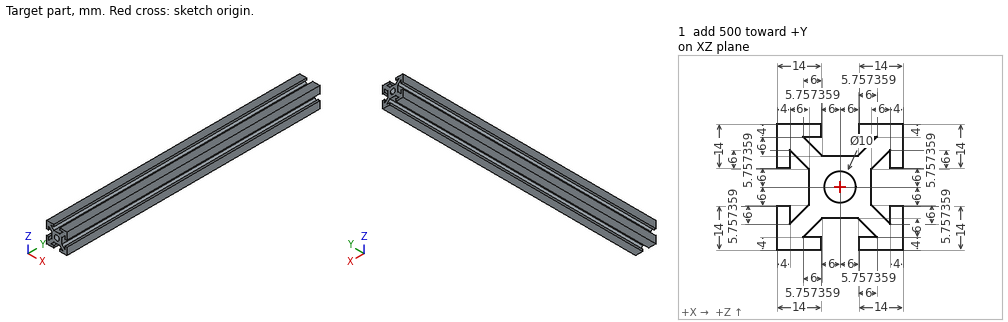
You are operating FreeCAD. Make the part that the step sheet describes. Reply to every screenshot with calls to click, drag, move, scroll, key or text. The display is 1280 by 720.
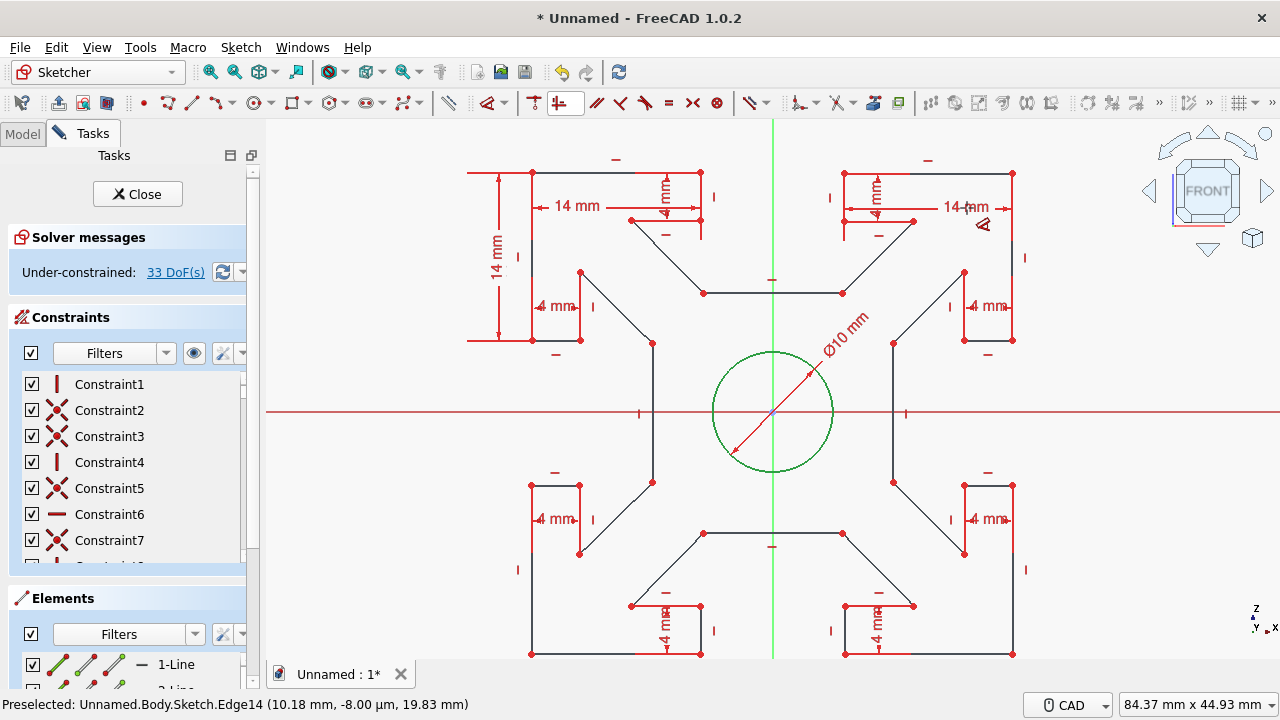
click(1012, 224)
click(1046, 257)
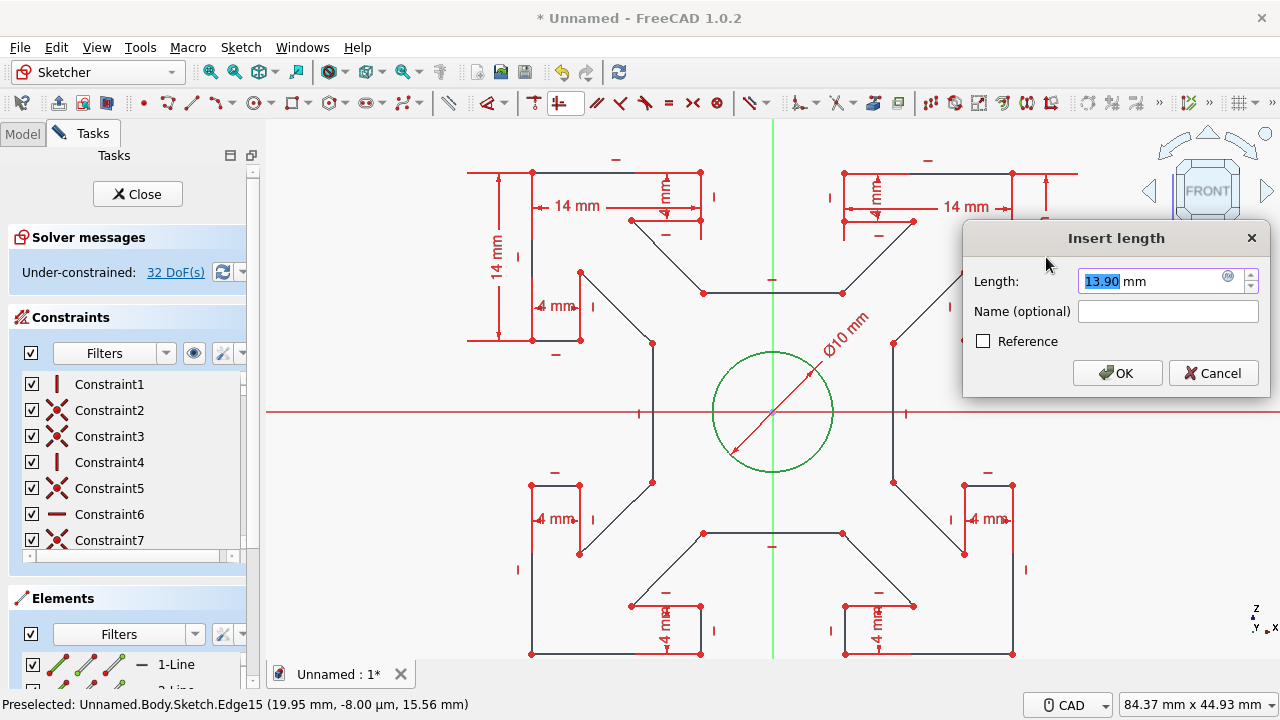
text(14)
key(Return)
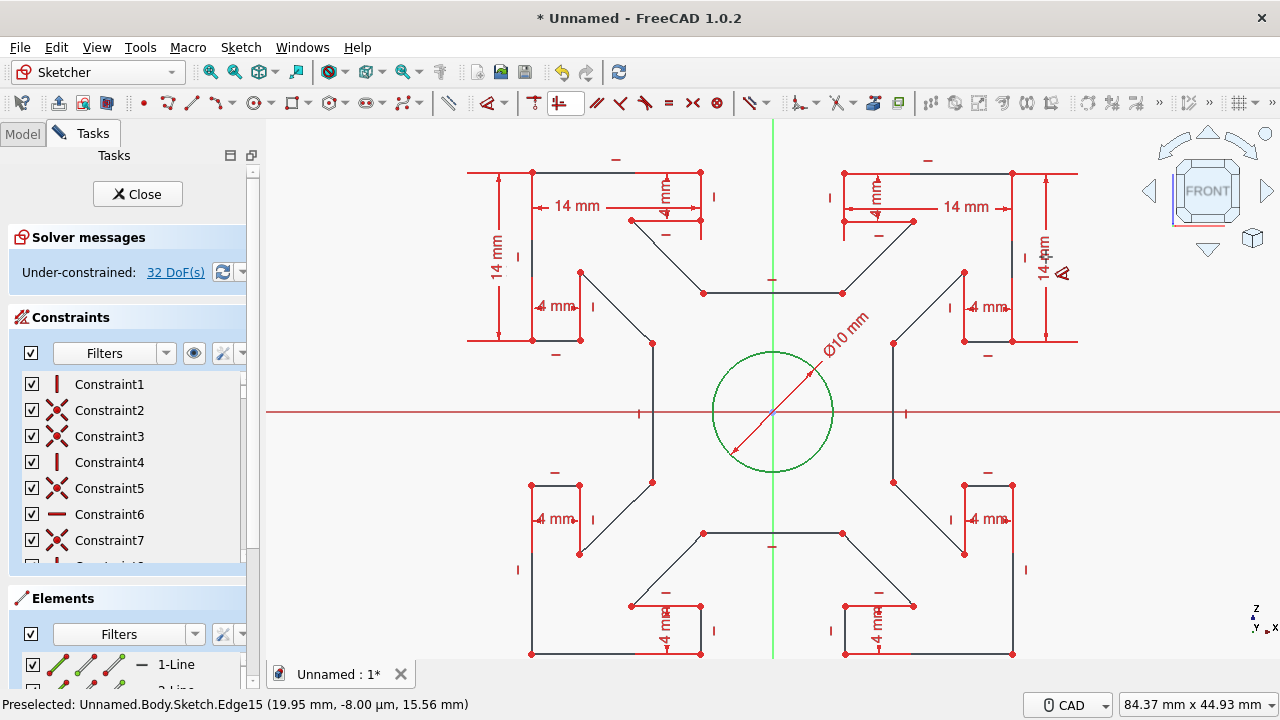
click(1013, 536)
click(1047, 558)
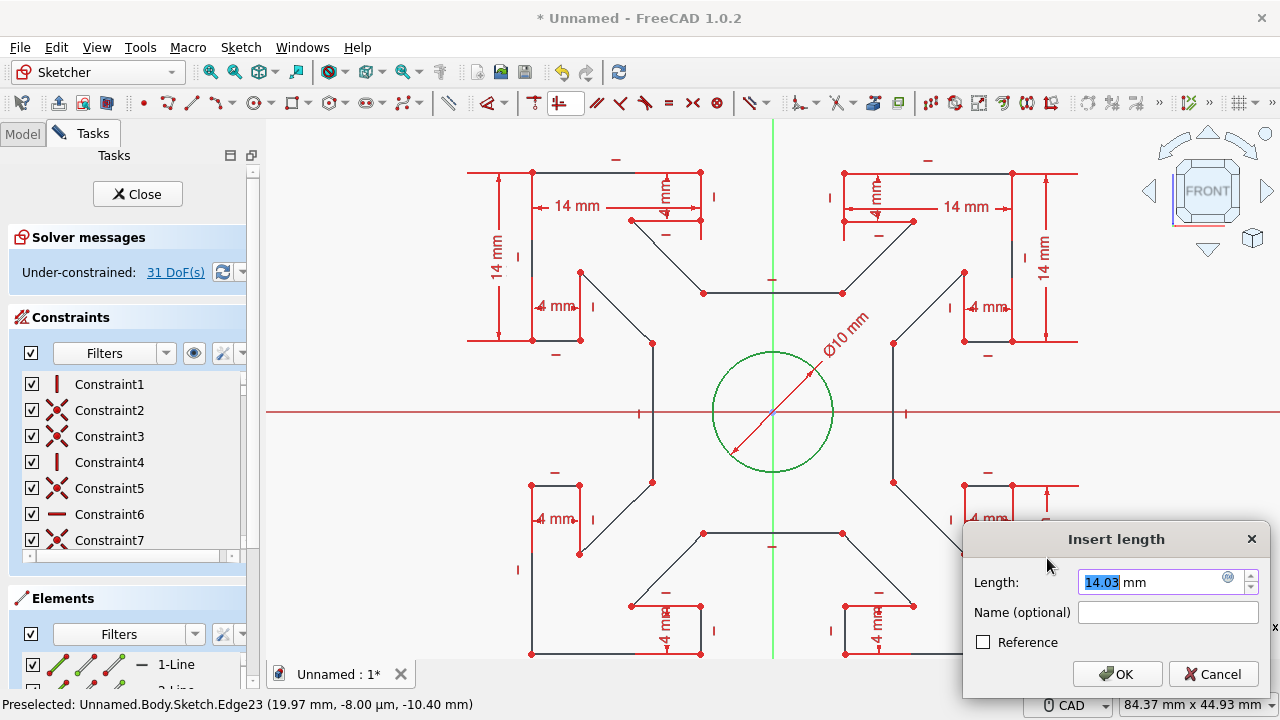
text(14)
key(Return)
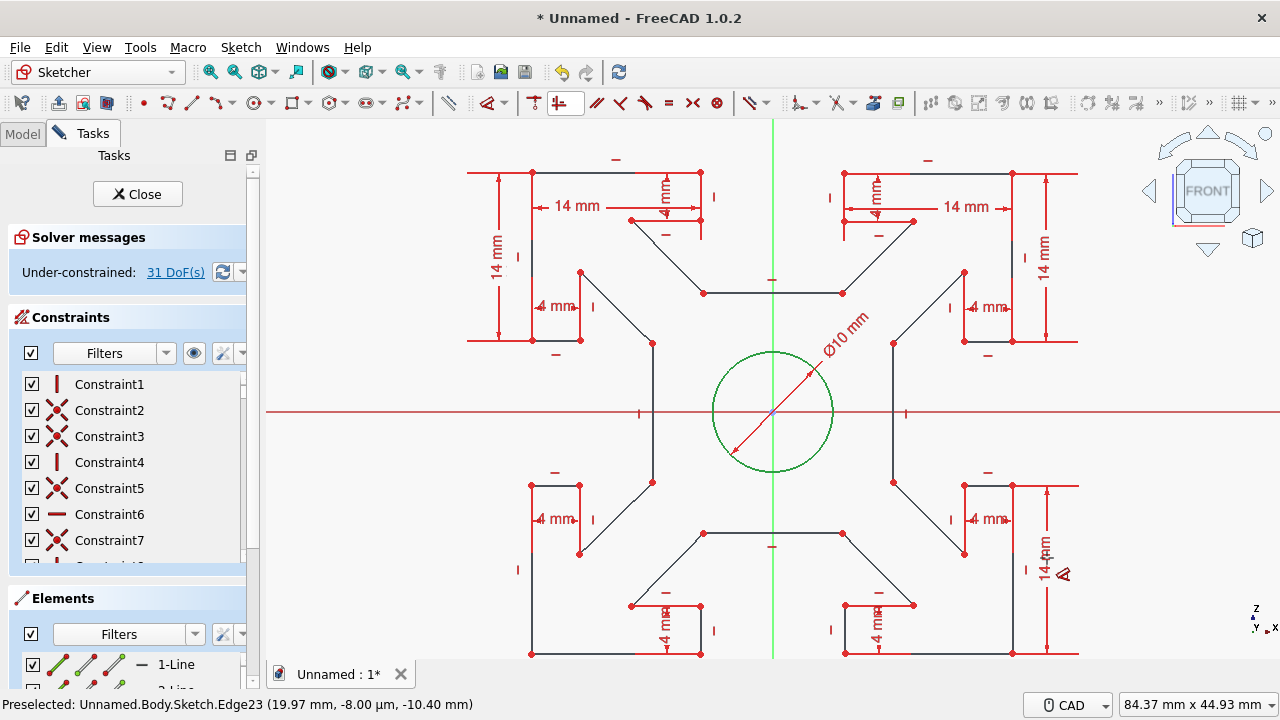
scroll(566, 342, down, 2)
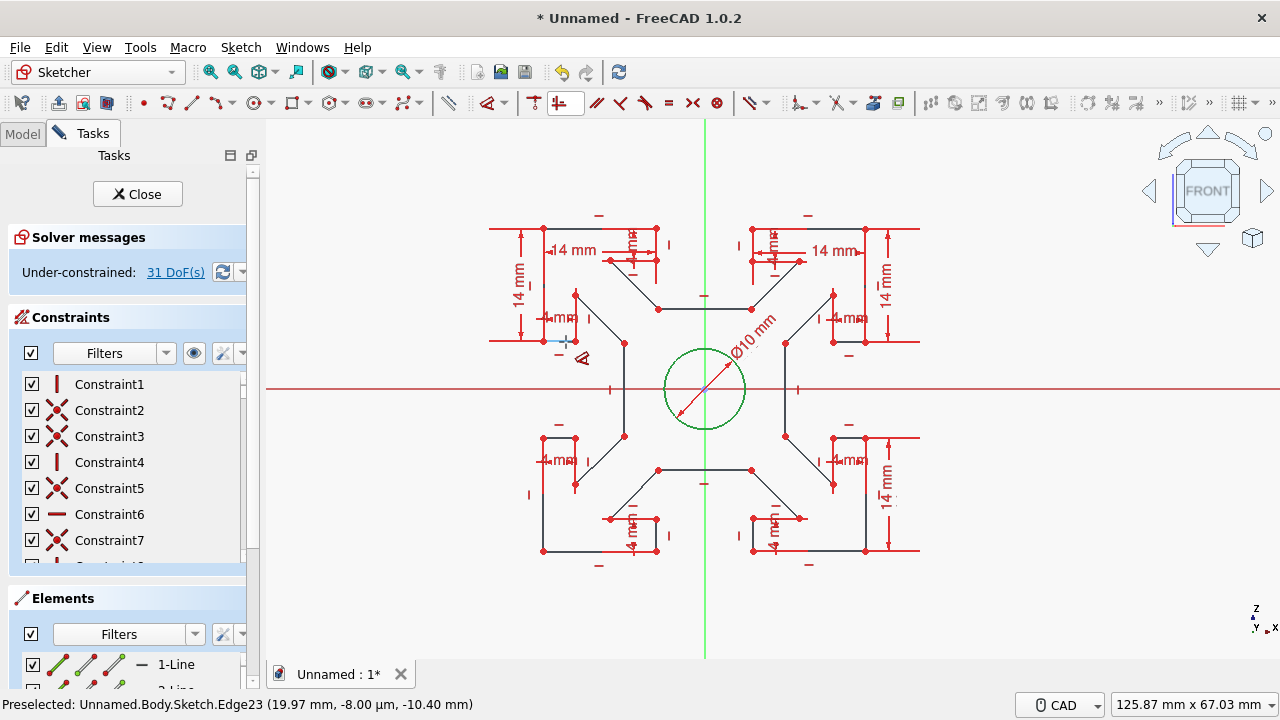
click(832, 551)
click(809, 585)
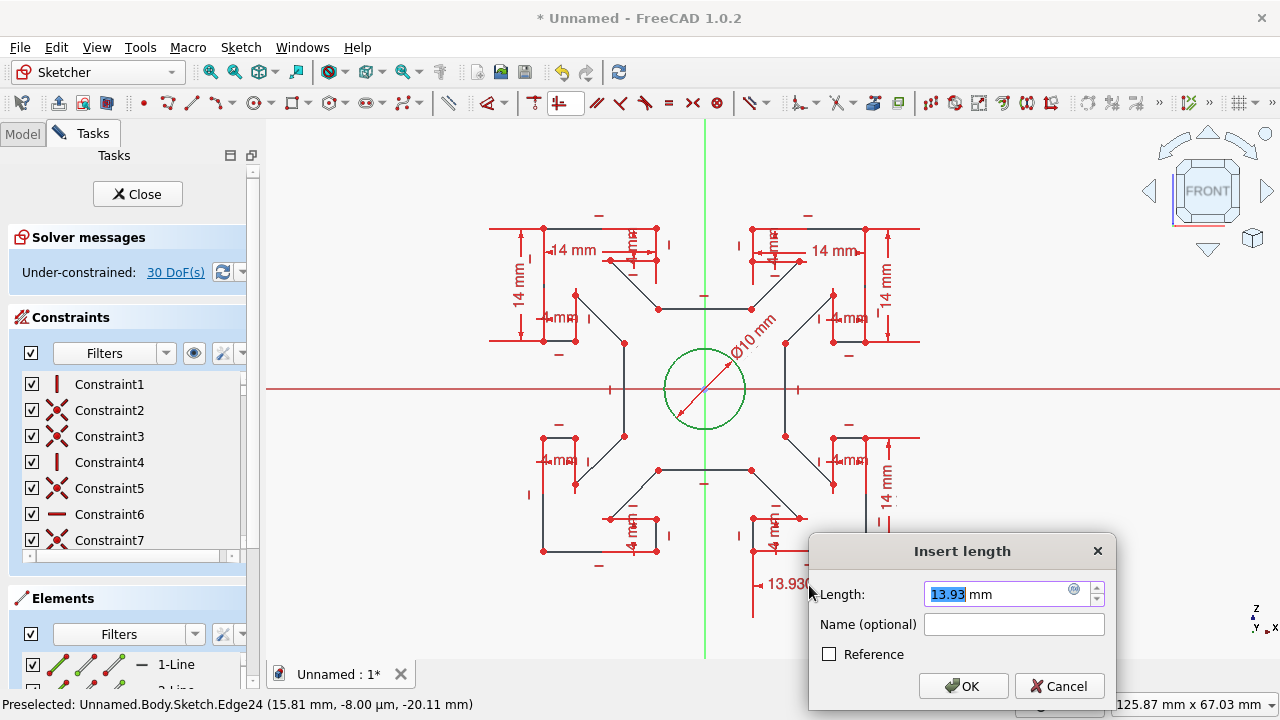
text(14)
key(Return)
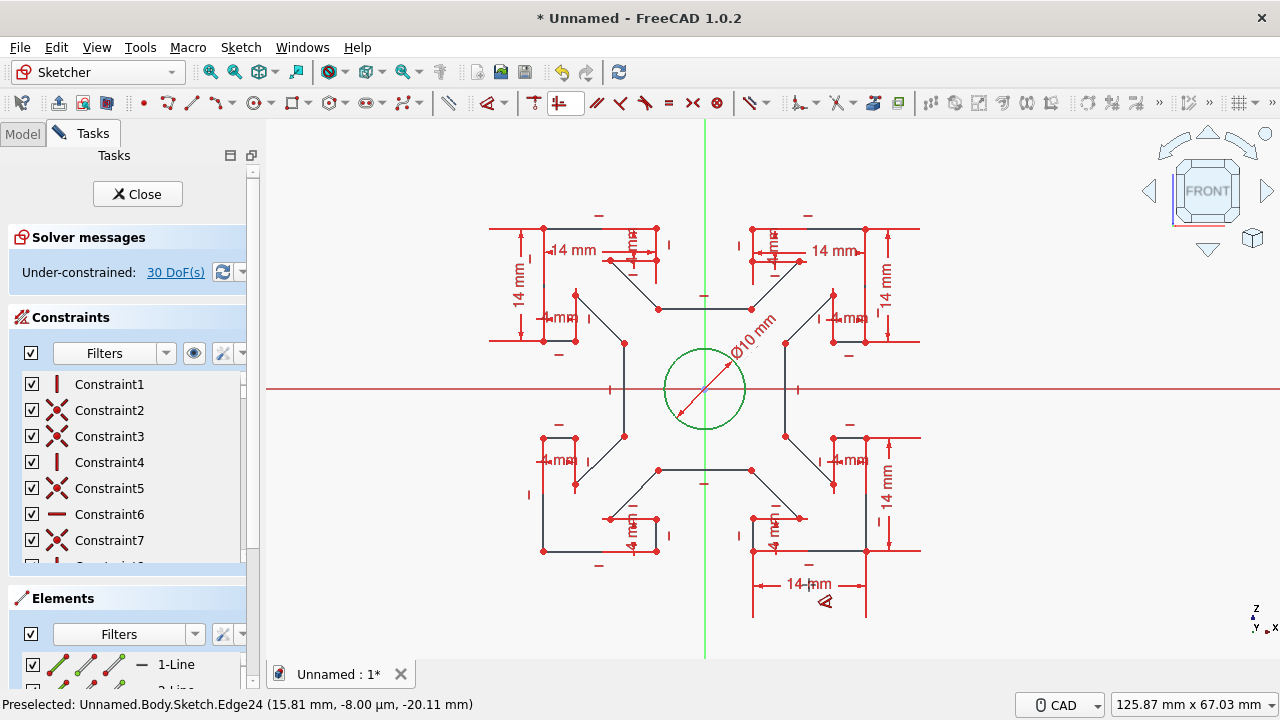
click(622, 552)
click(600, 586)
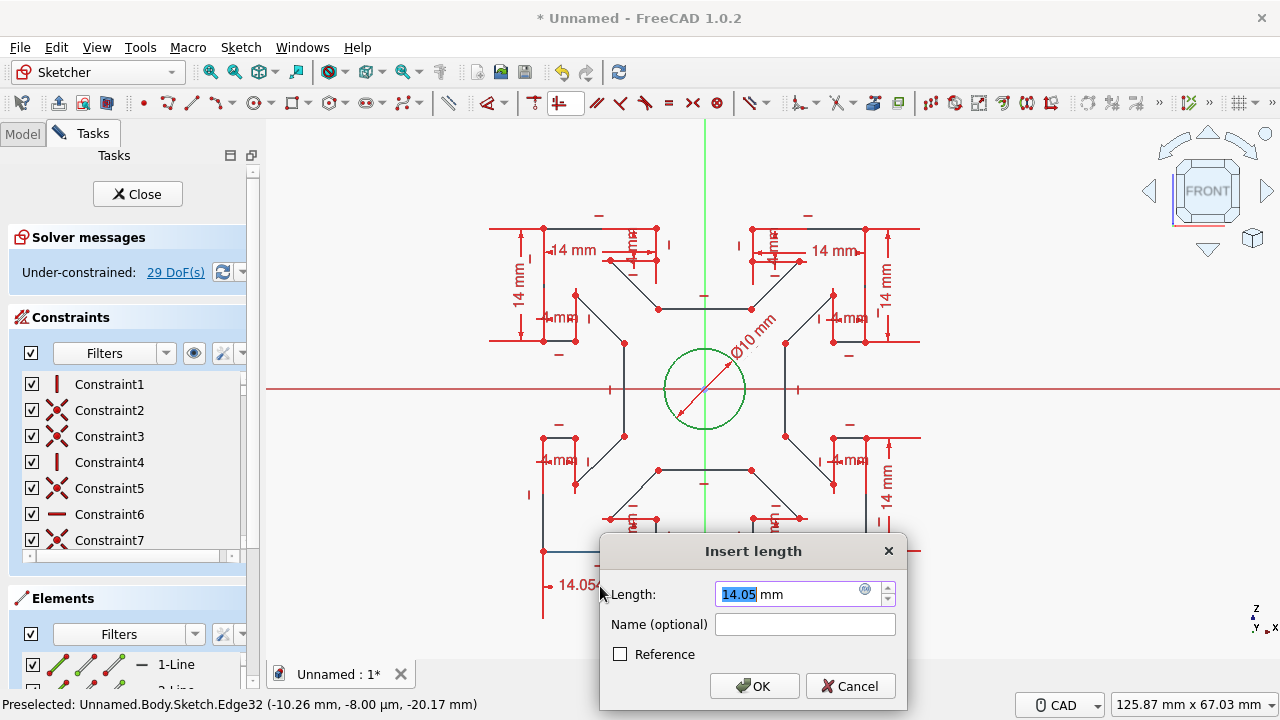
text(14)
key(Return)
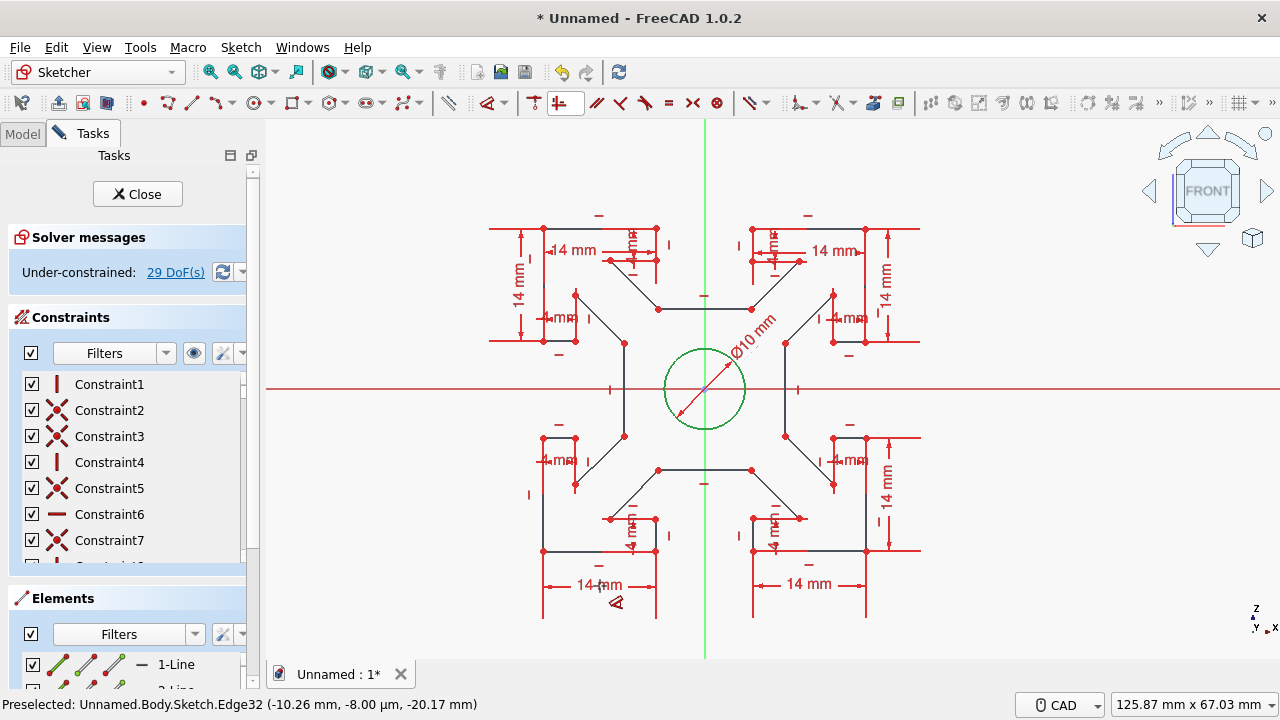
click(543, 518)
click(509, 495)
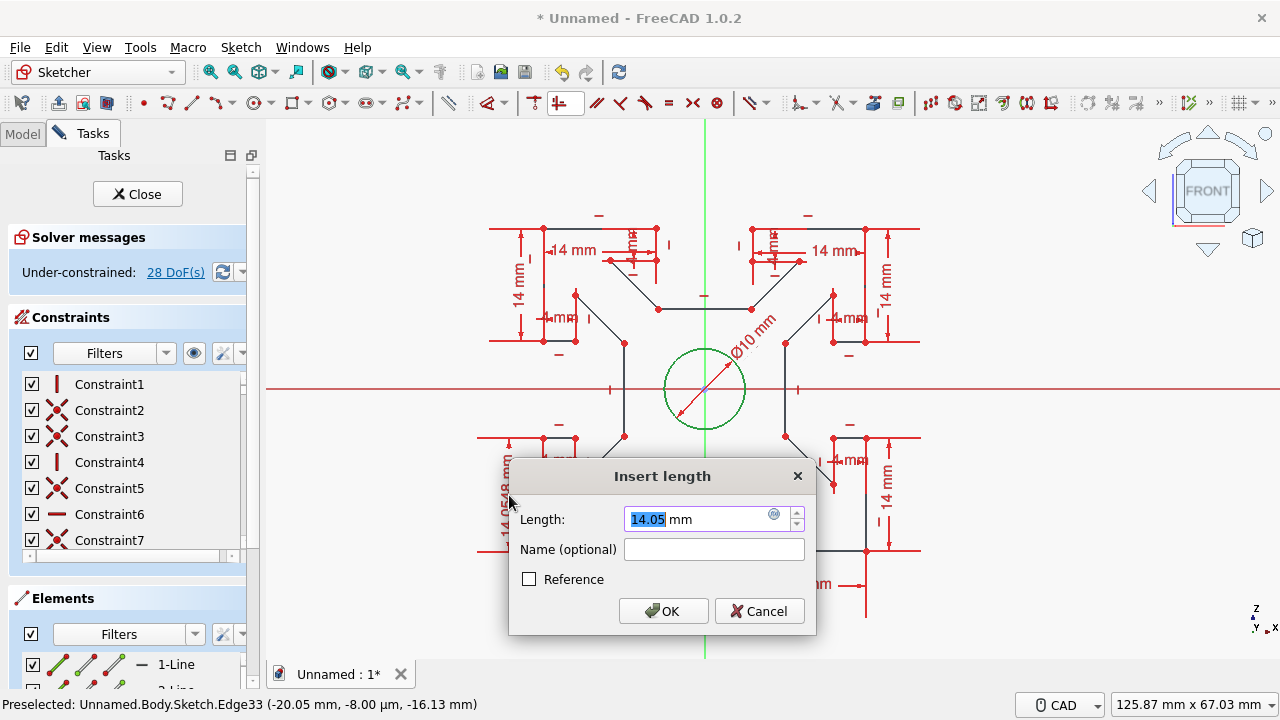
text(14)
key(Return)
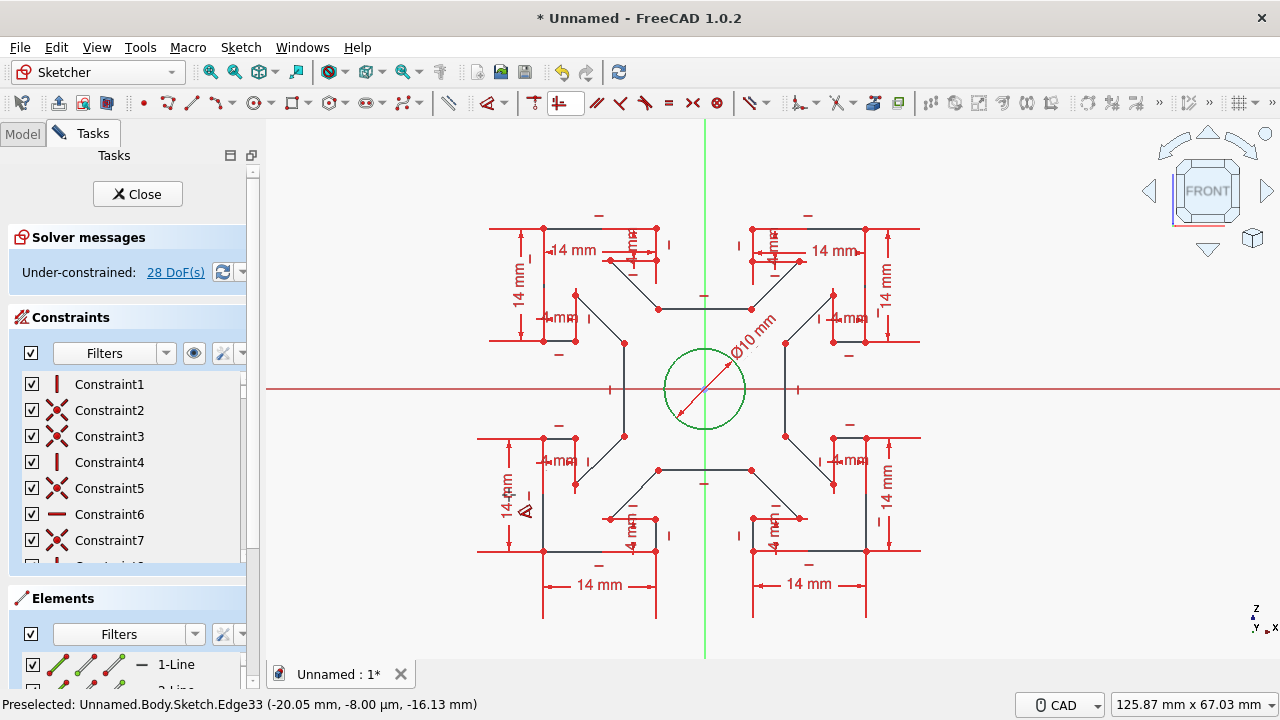
click(576, 341)
click(542, 365)